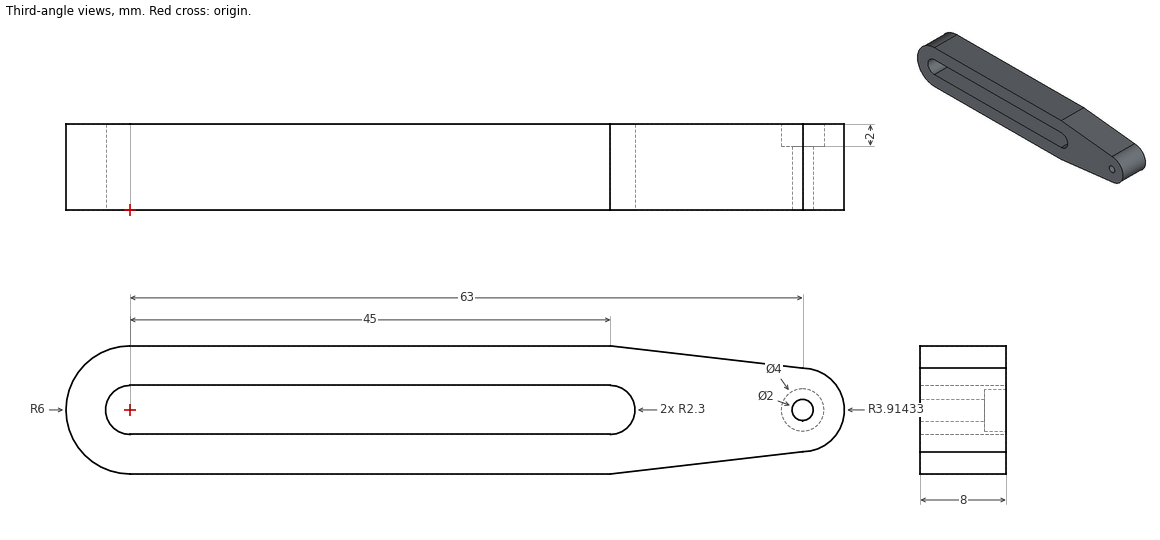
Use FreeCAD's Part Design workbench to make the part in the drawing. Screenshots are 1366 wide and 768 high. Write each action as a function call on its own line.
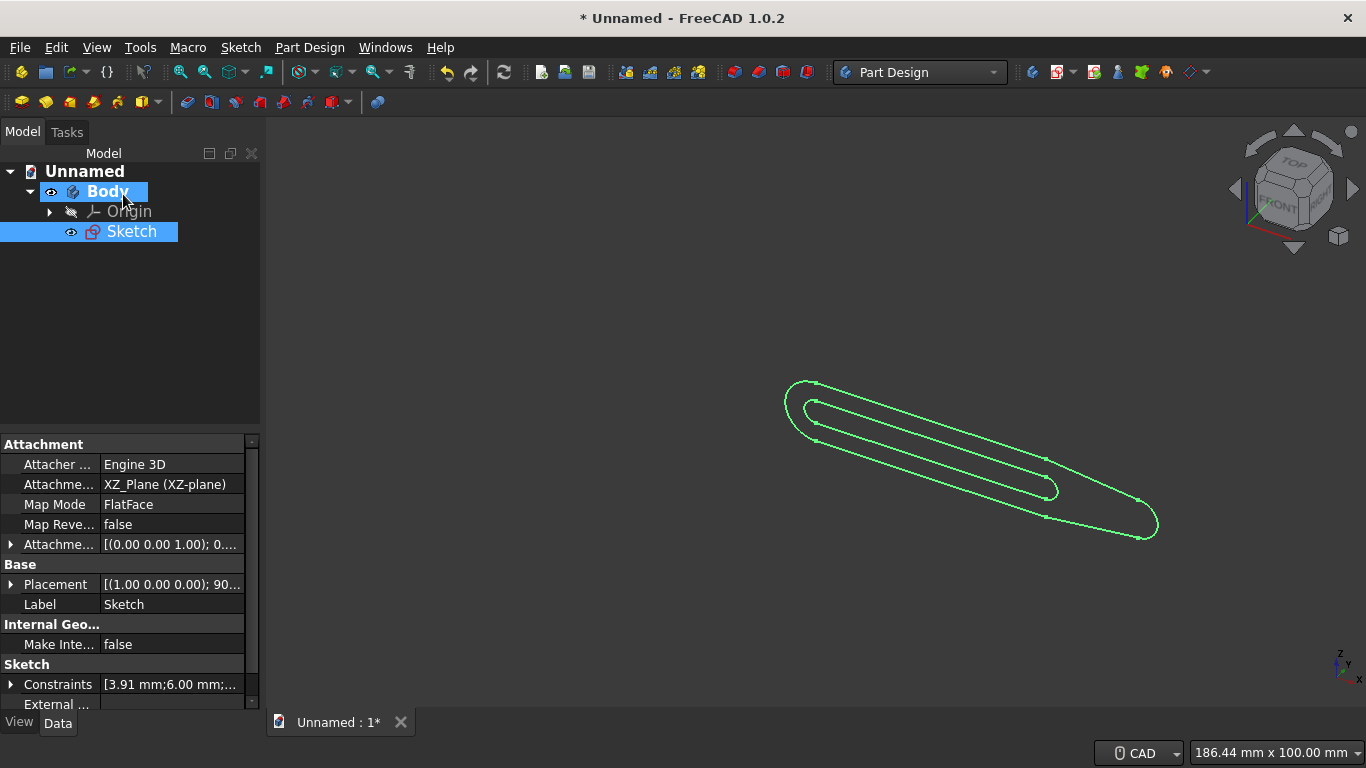
click(22, 102)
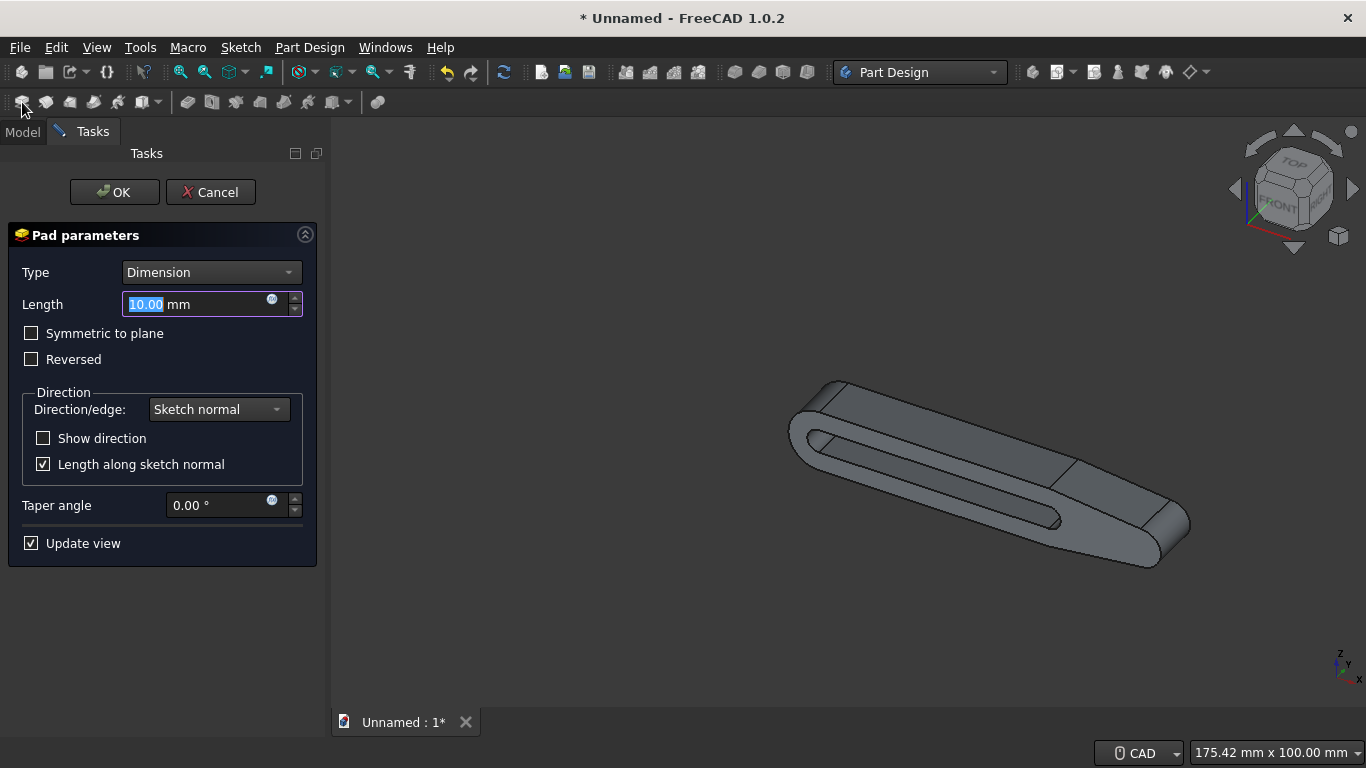
text(8)
key(Tab)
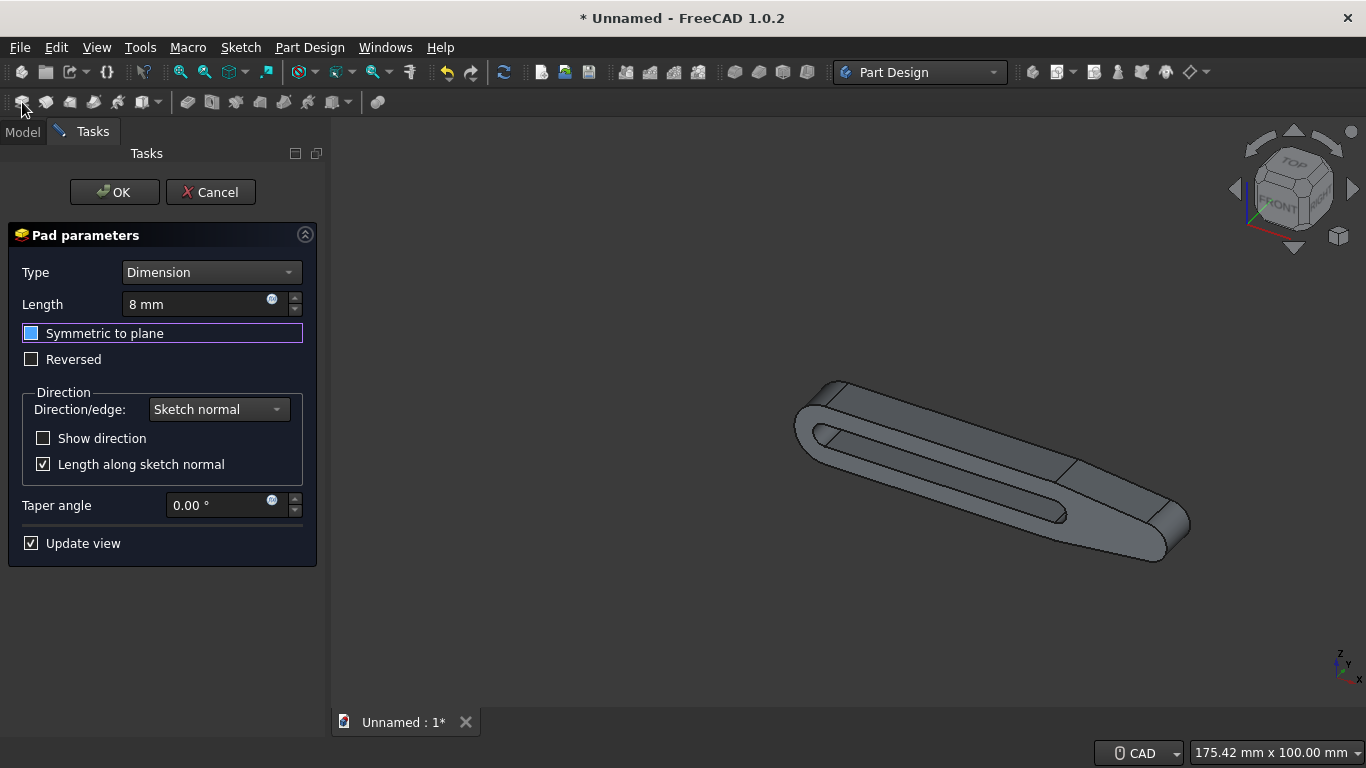
click(30, 359)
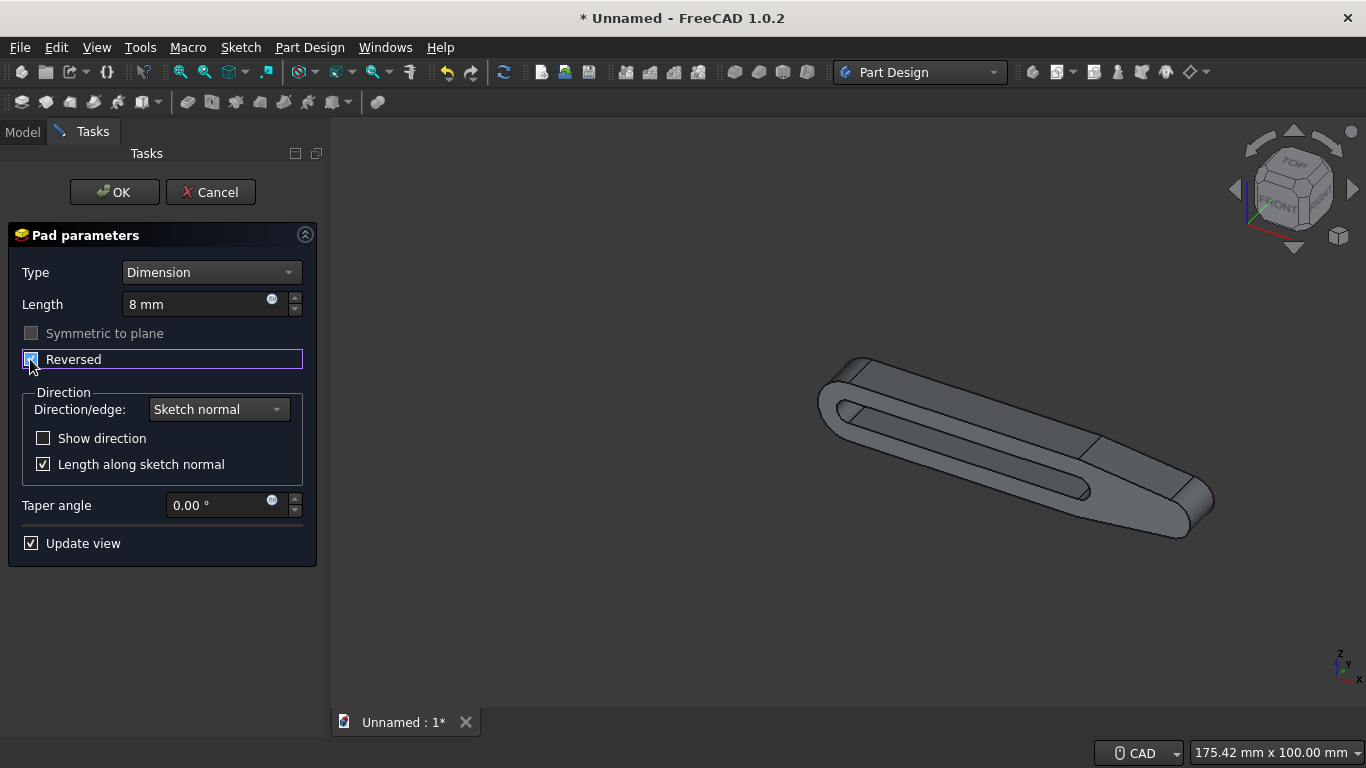
click(115, 192)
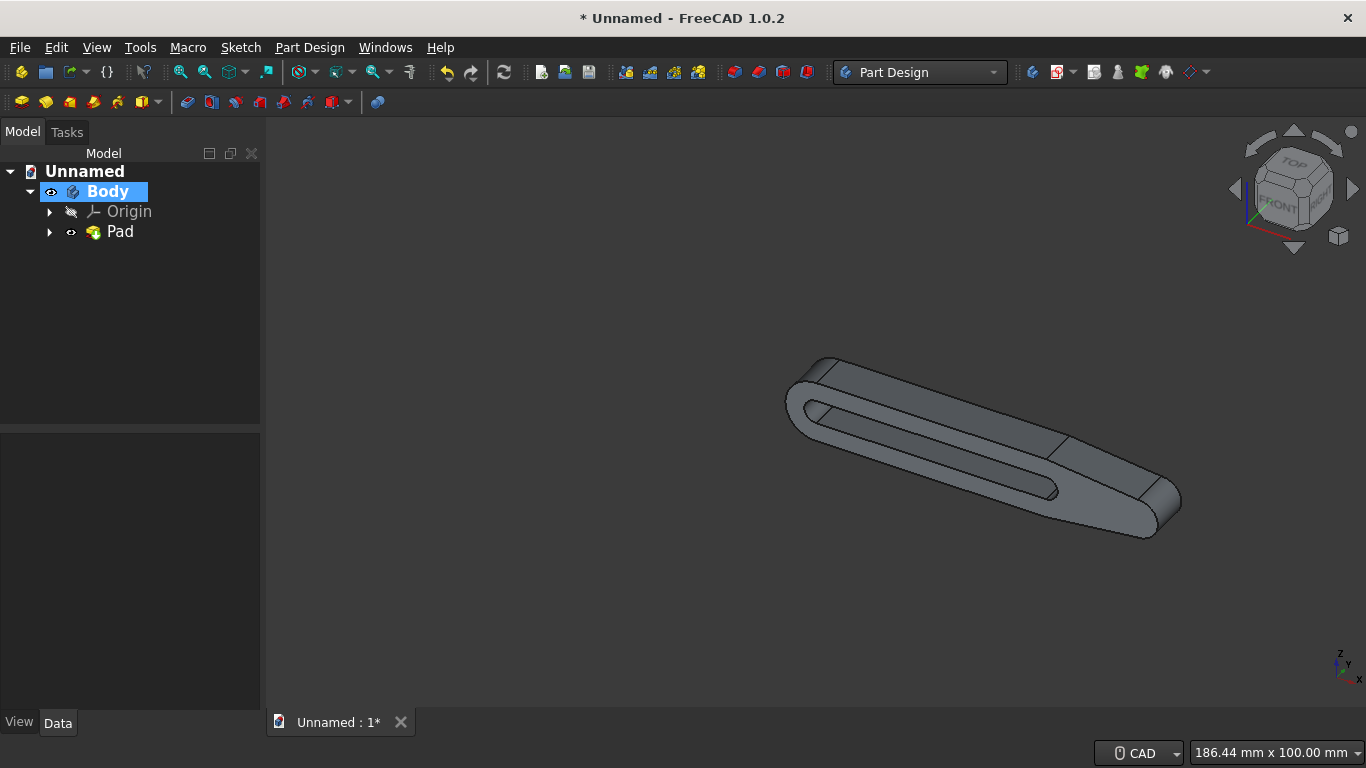
click(182, 72)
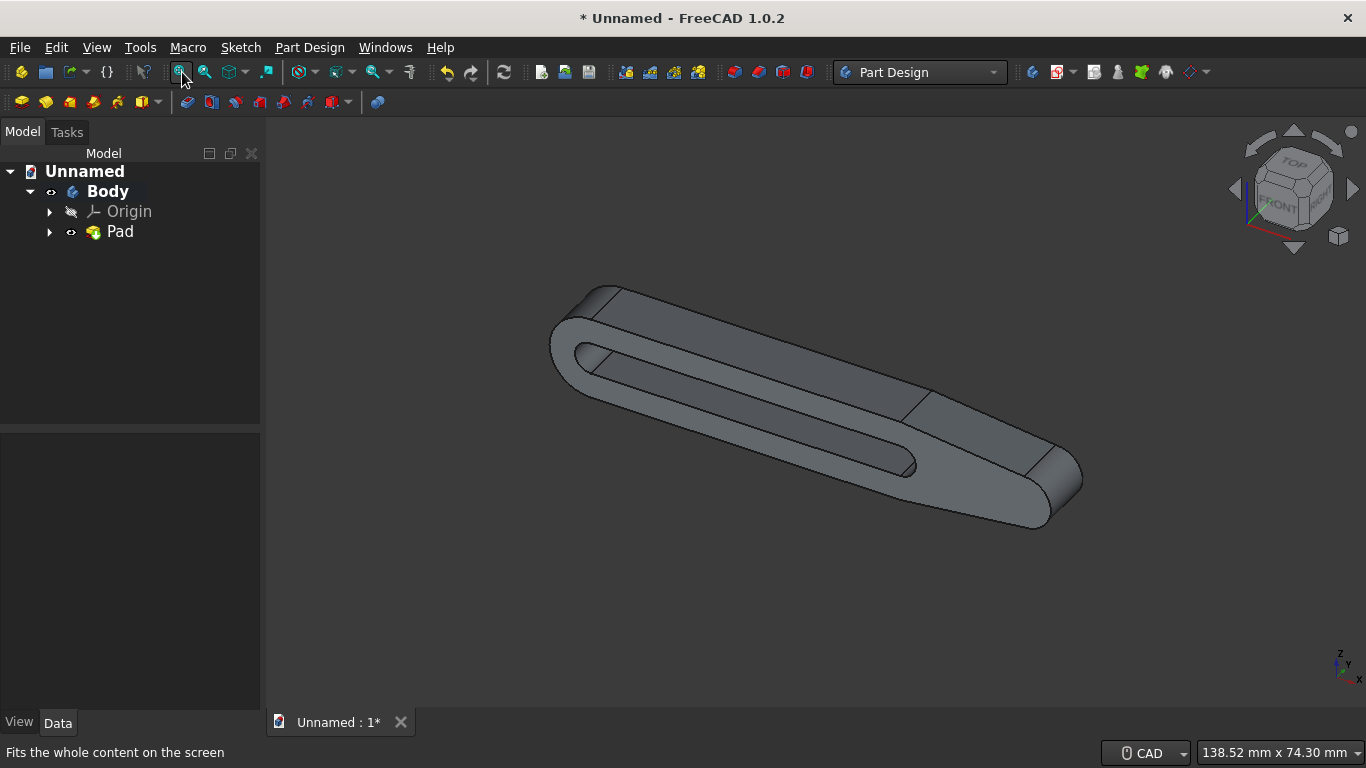
key(4)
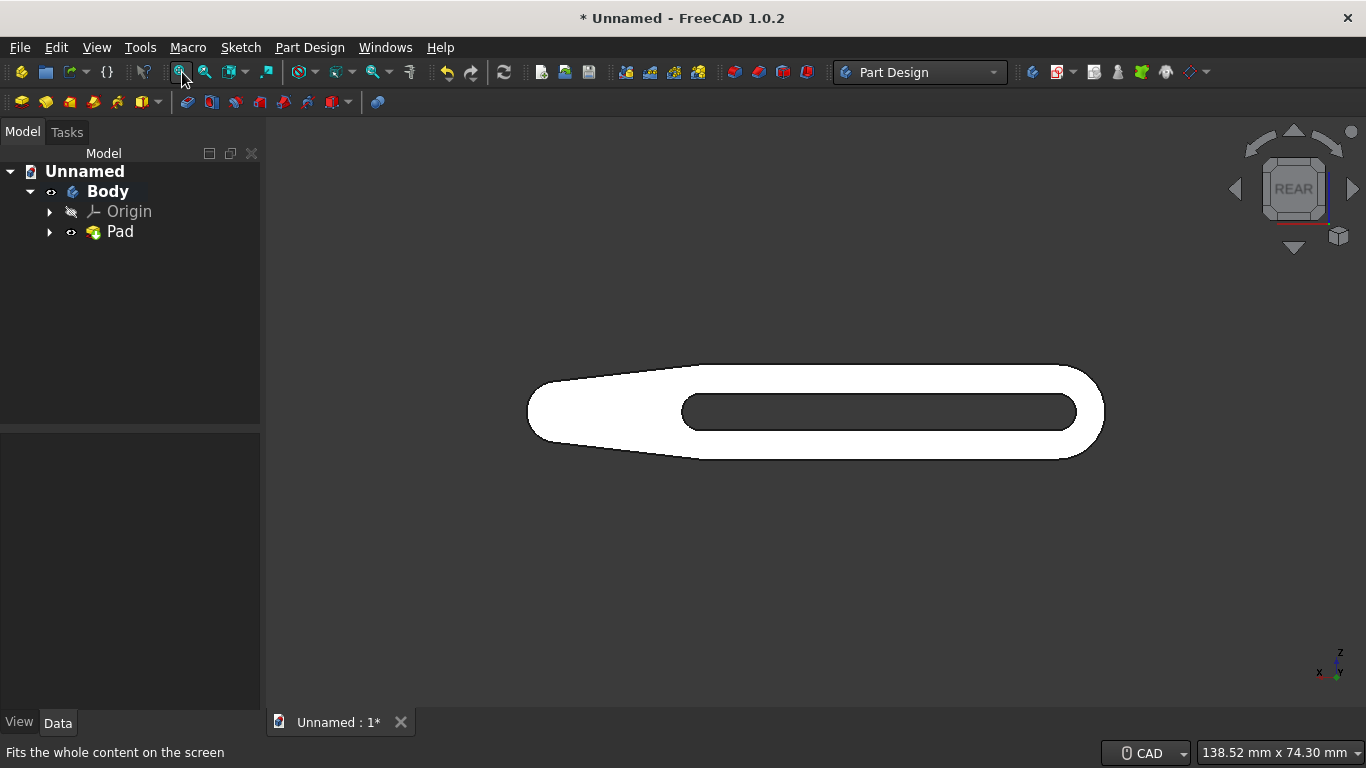
click(568, 411)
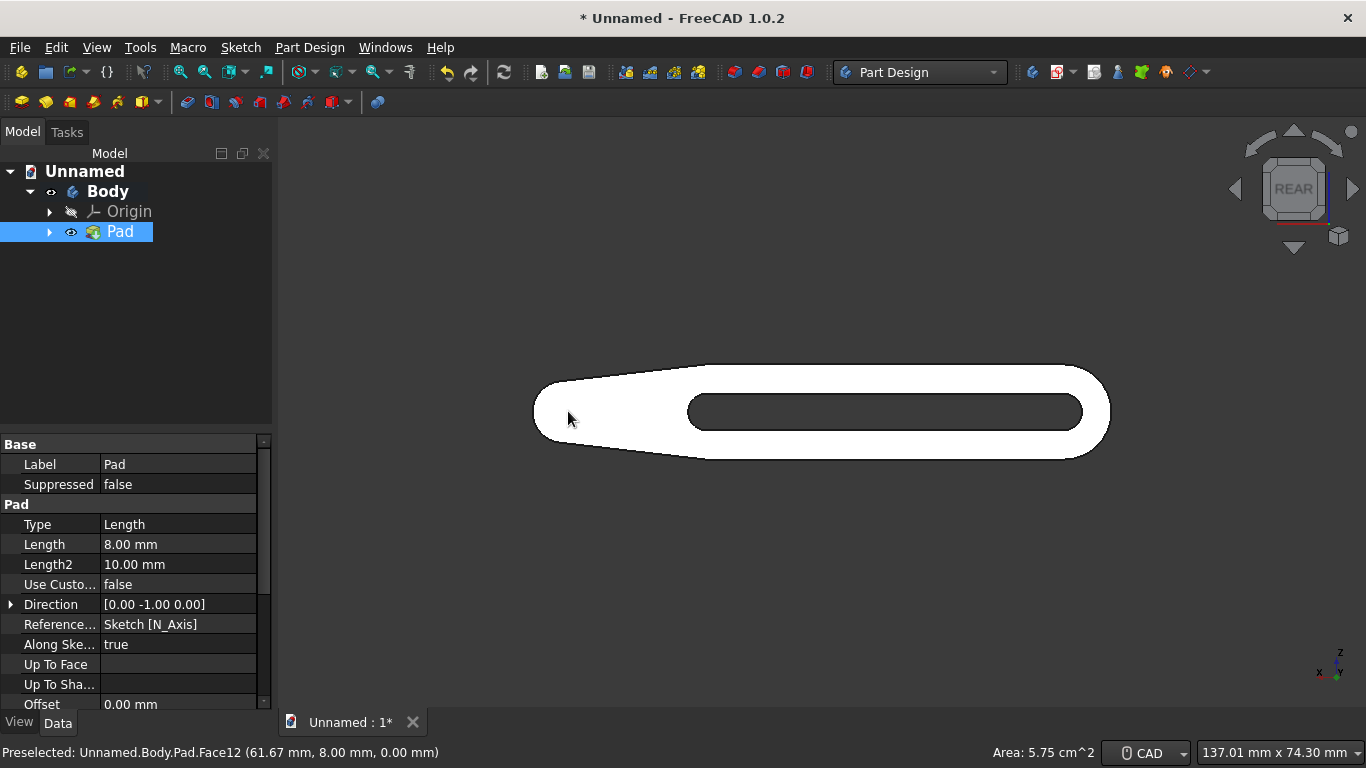
click(1058, 72)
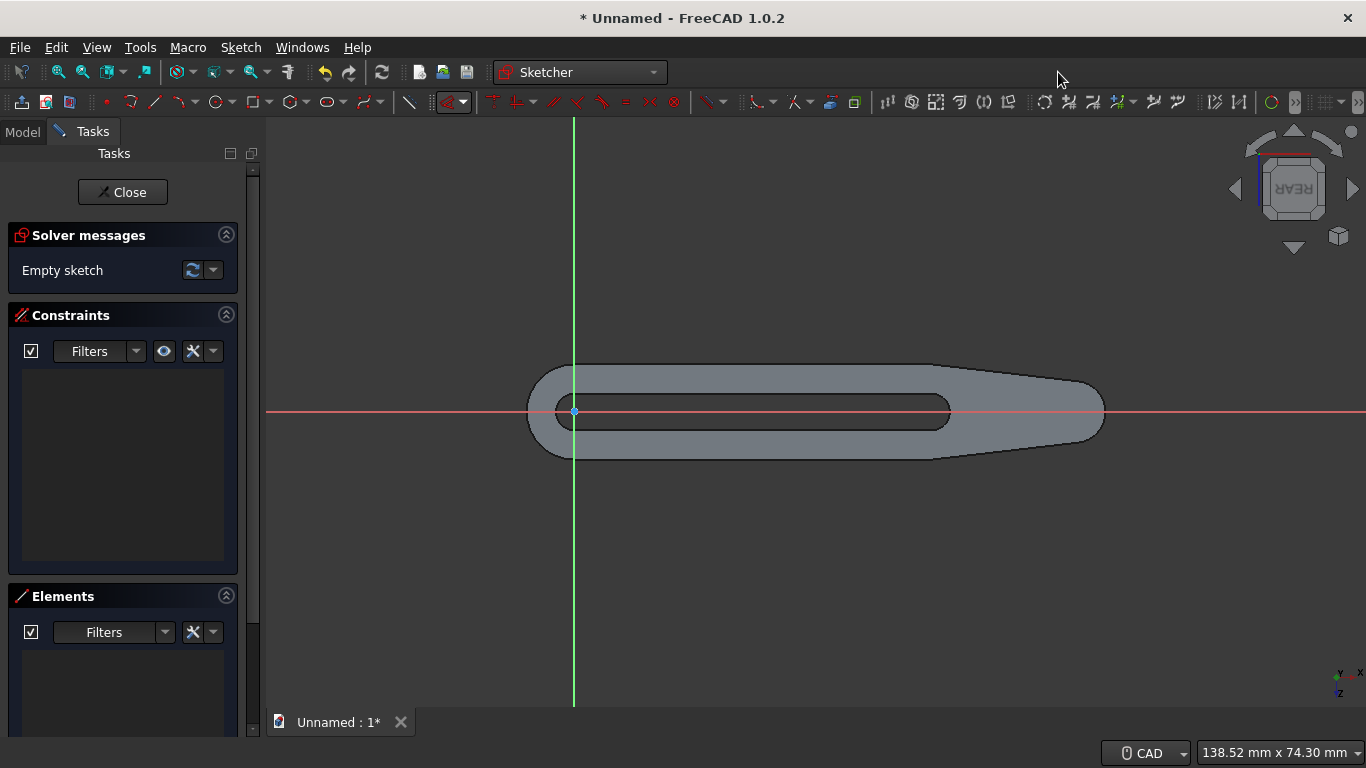
scroll(1107, 412, up, 12)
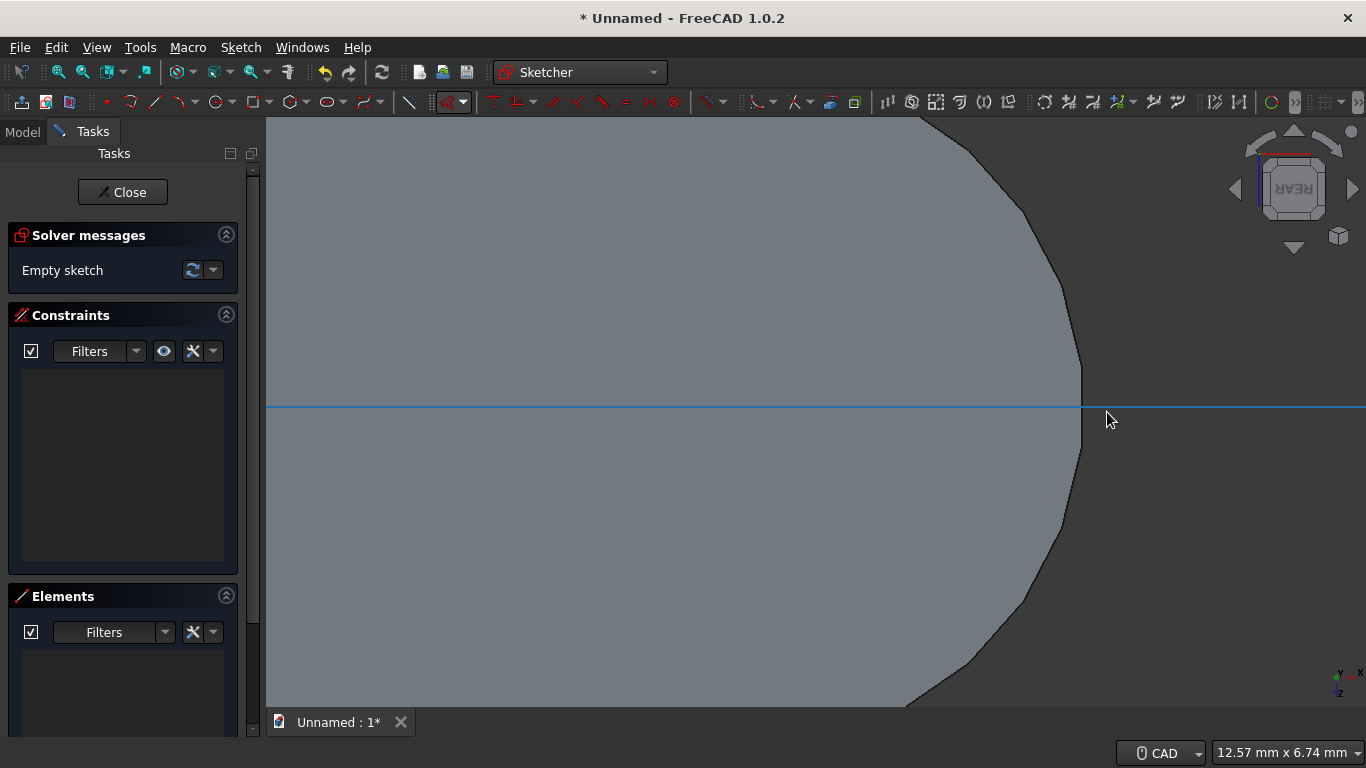
click(216, 102)